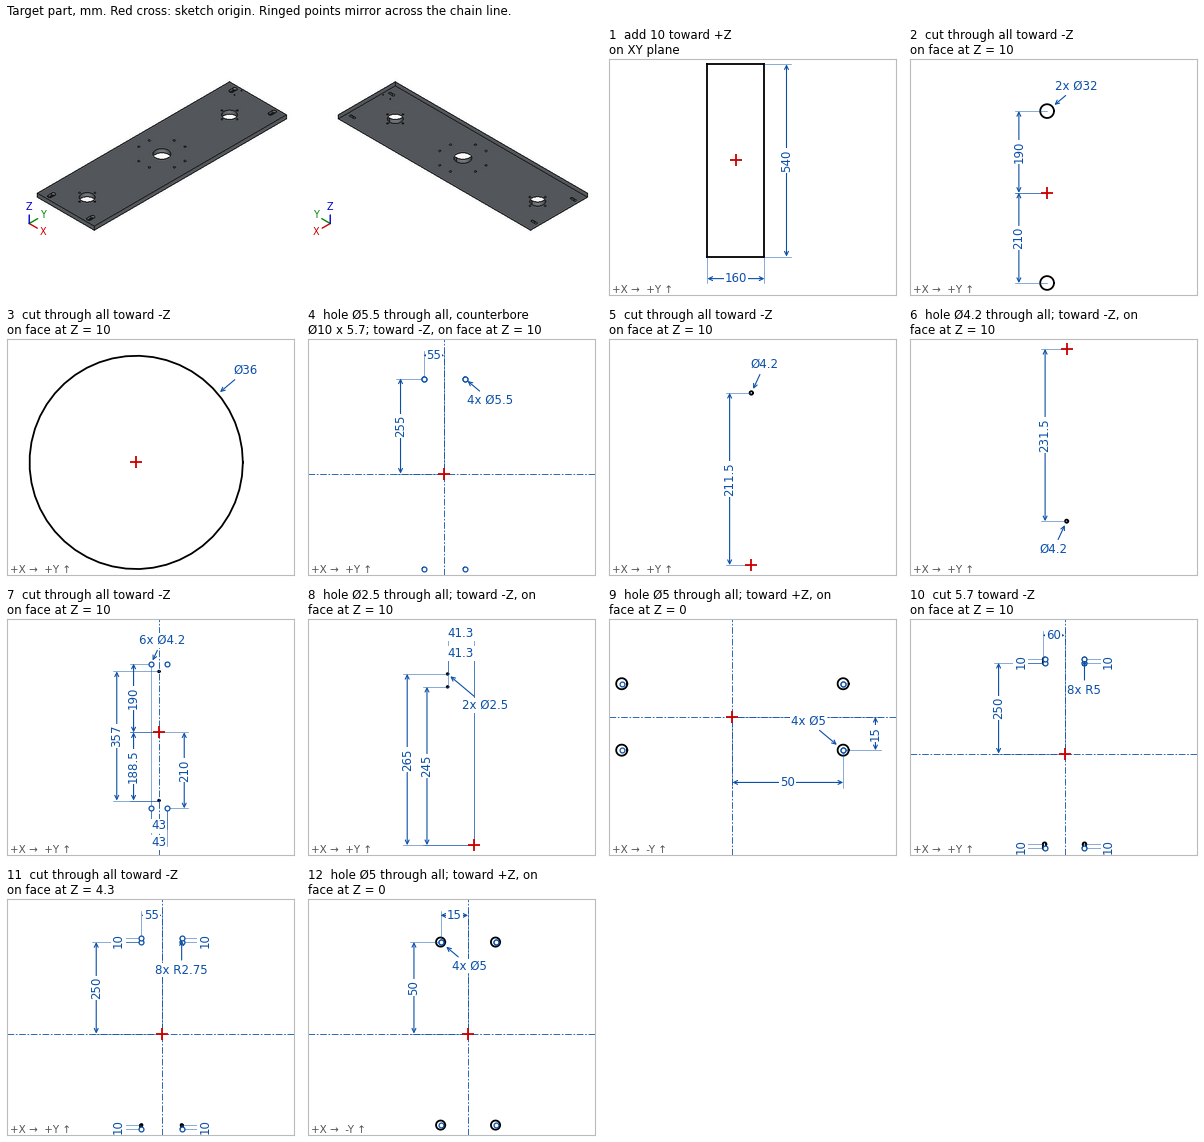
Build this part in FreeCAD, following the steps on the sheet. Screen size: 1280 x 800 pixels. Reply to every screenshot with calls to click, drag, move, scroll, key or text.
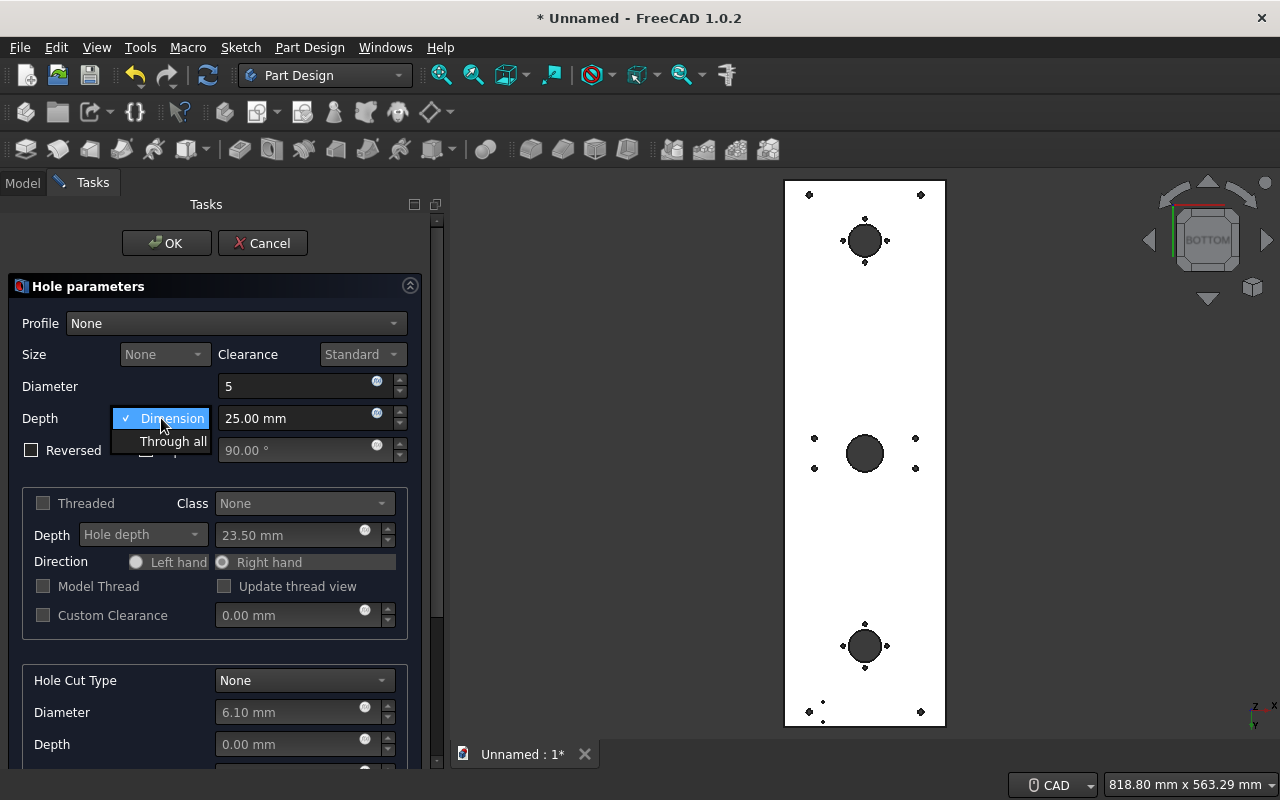
click(160, 442)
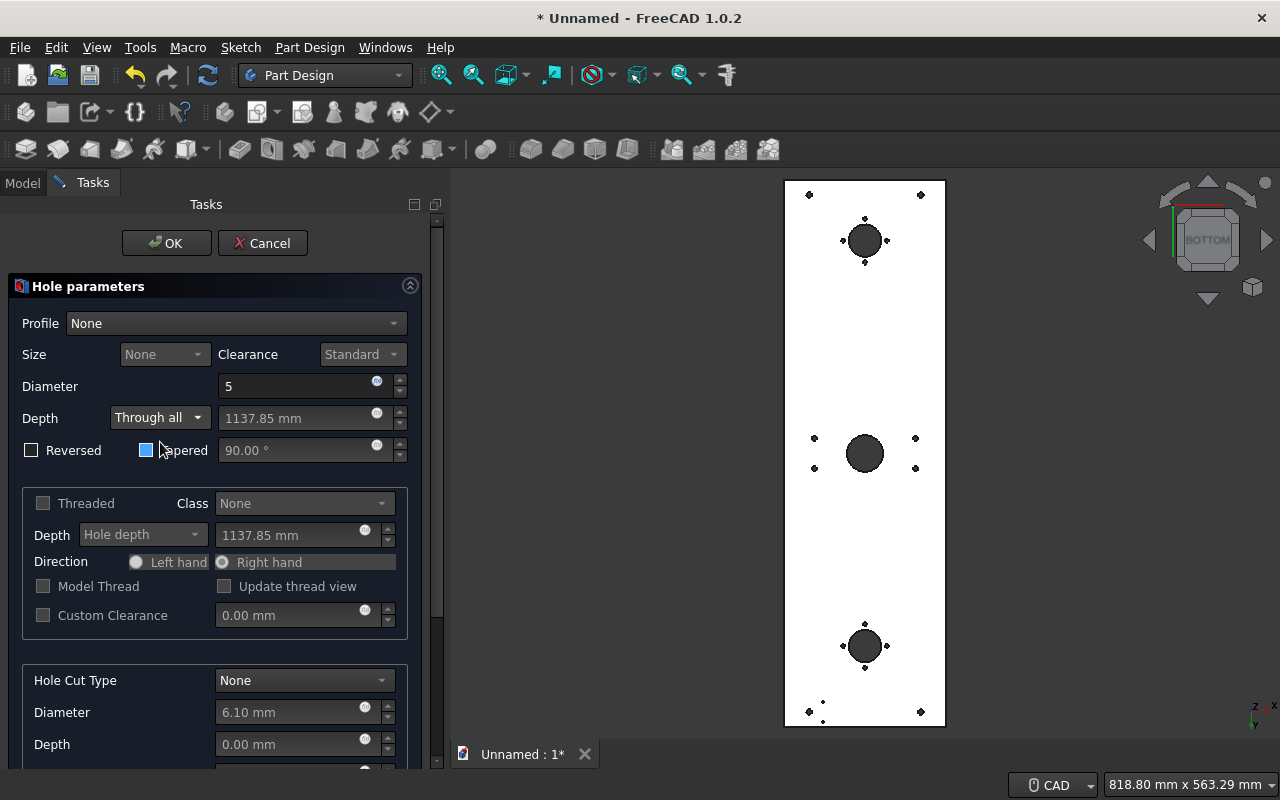
click(167, 243)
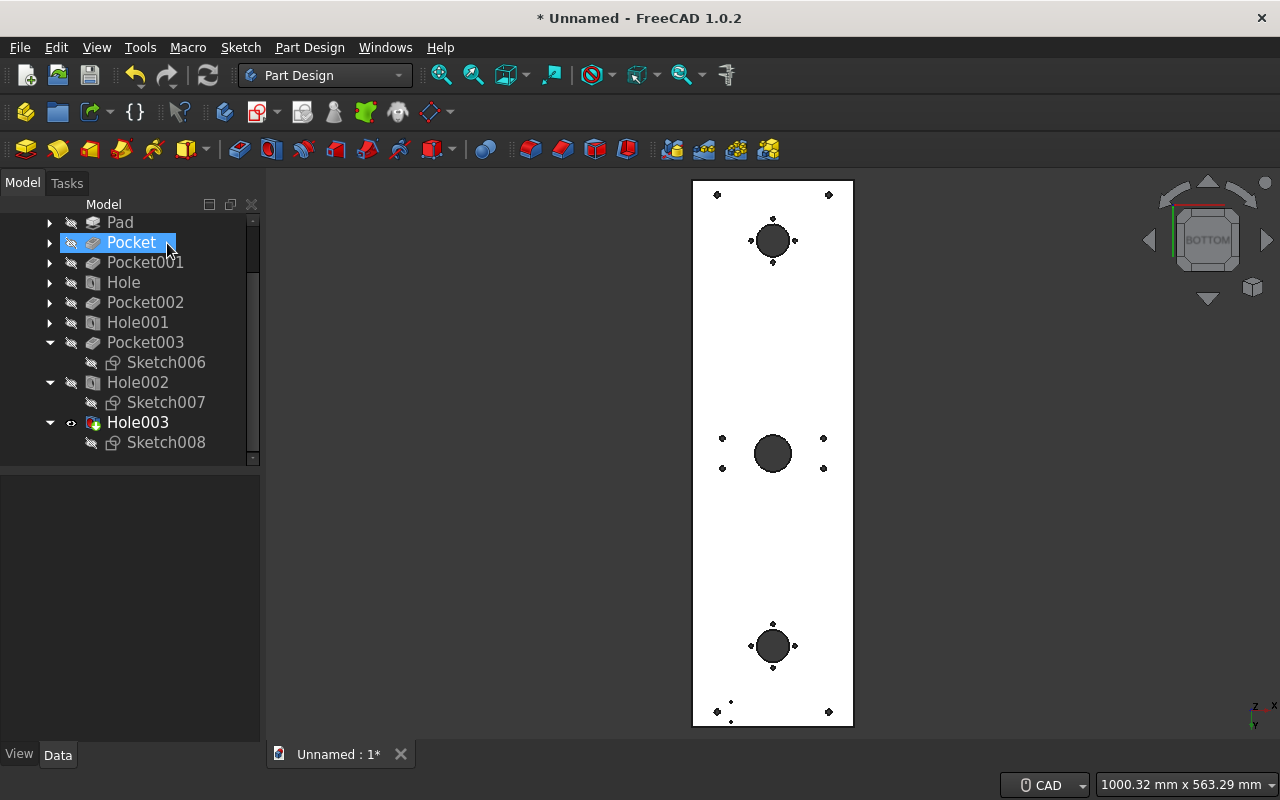
key(0)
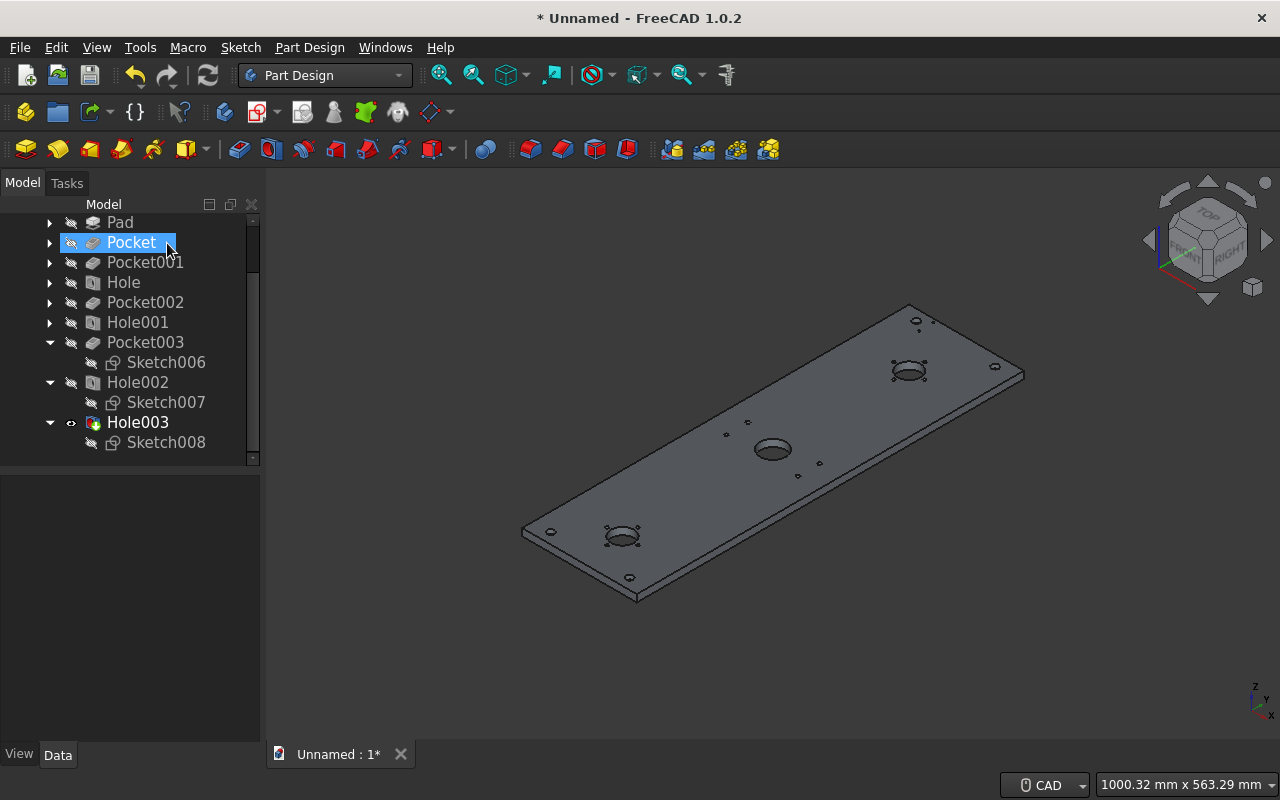
click(828, 416)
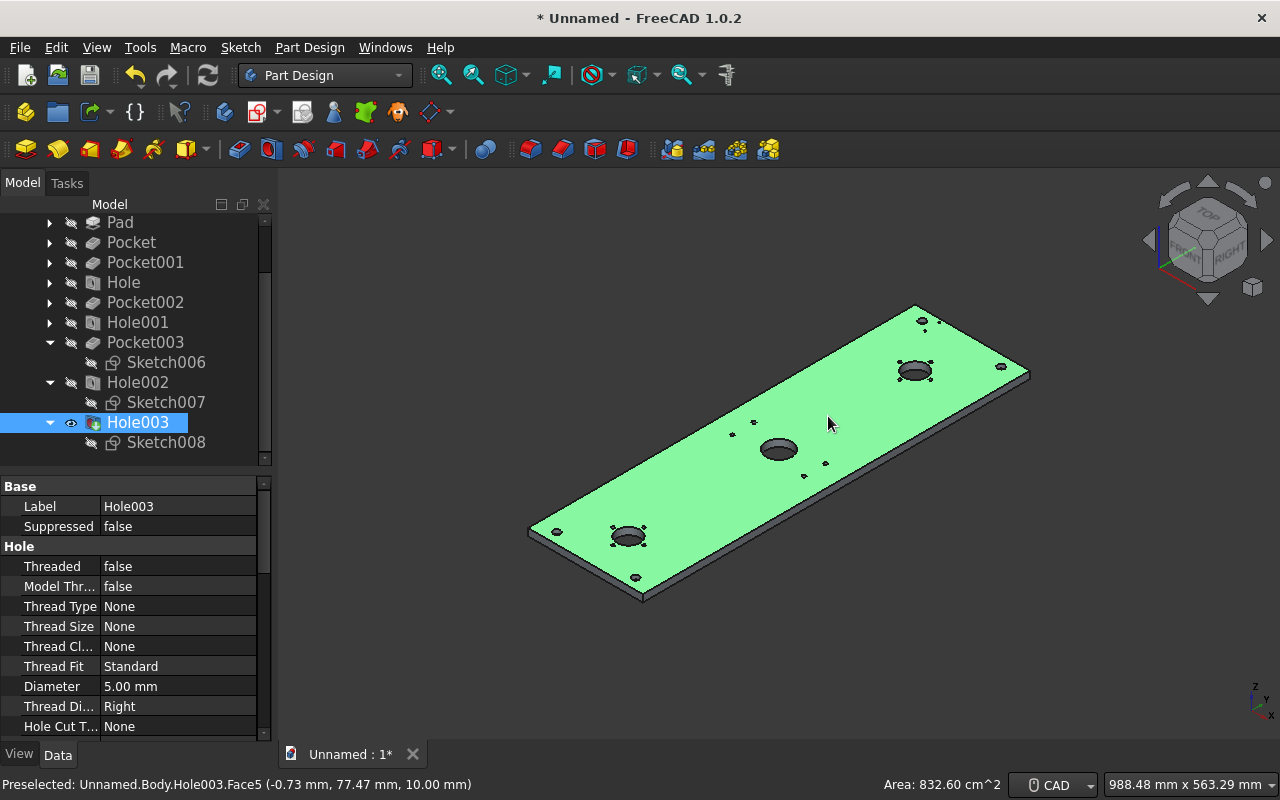
click(258, 112)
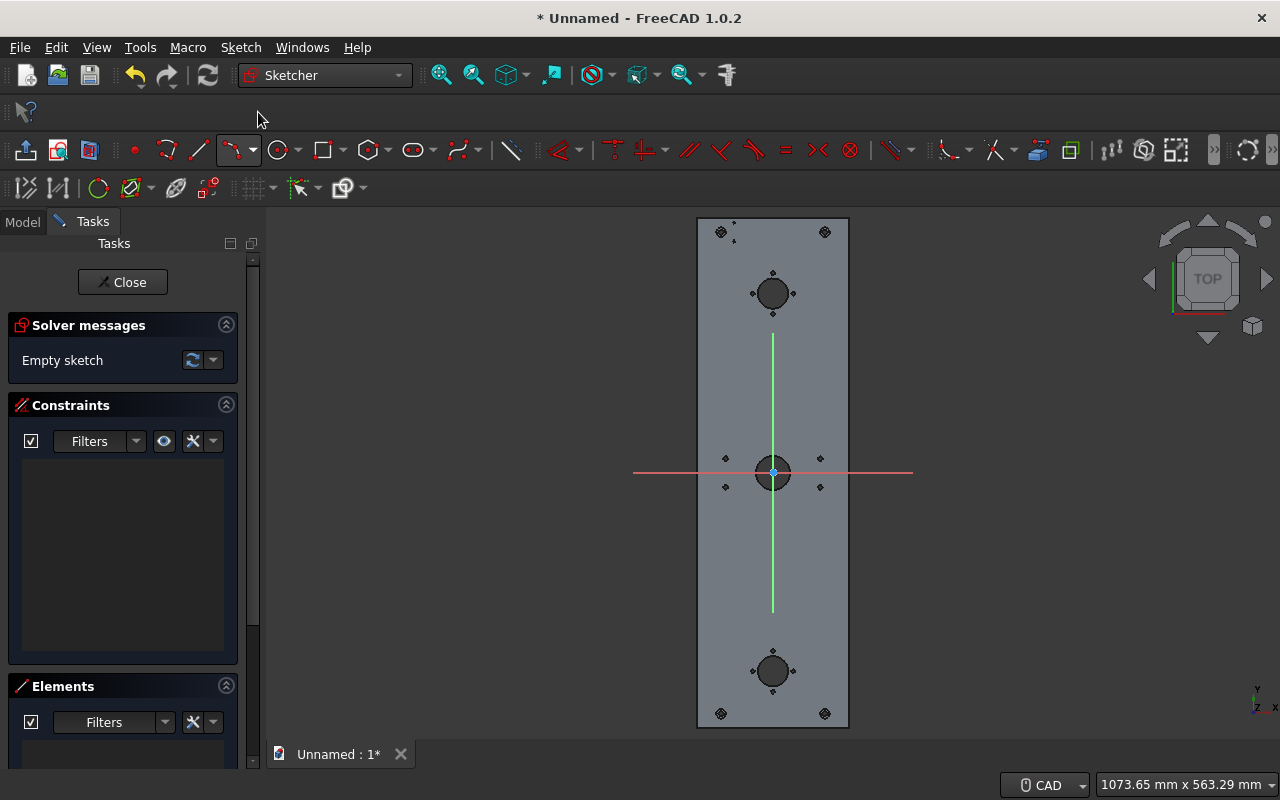
scroll(565, 473, down, 2)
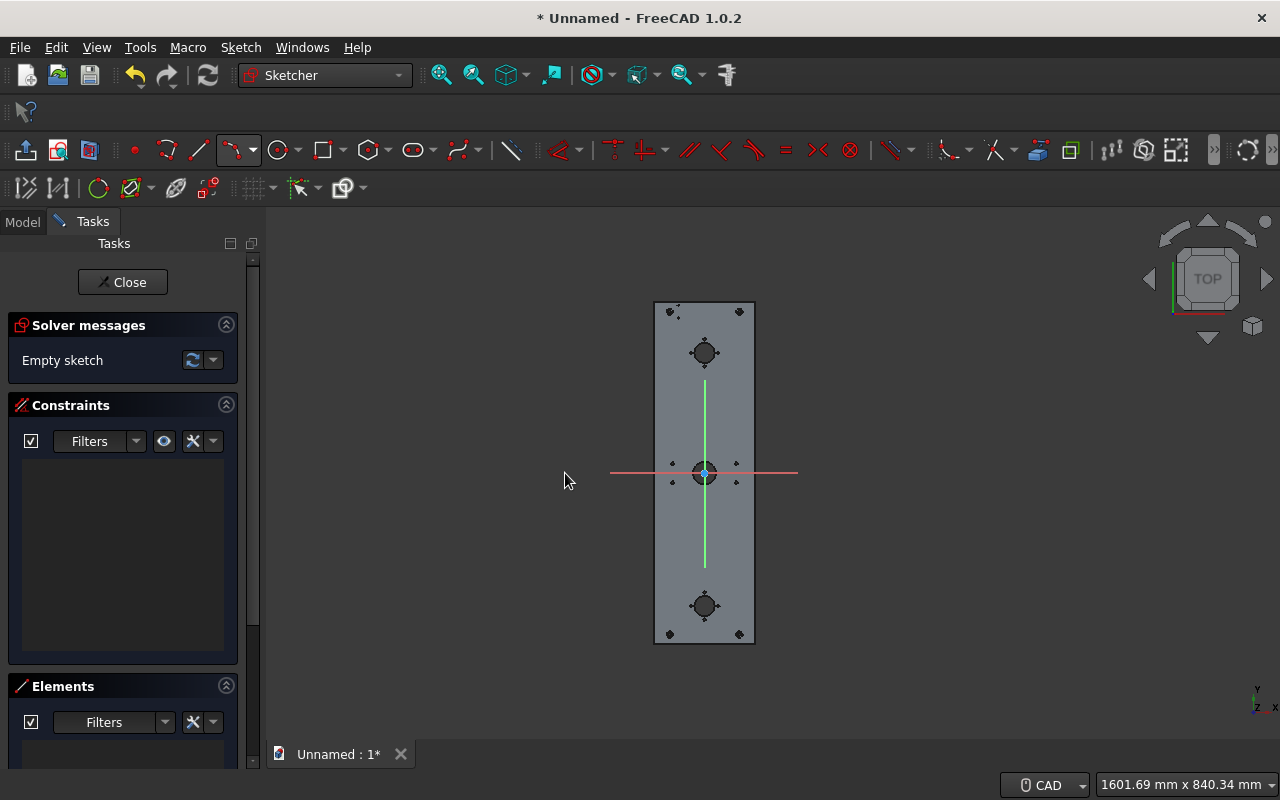
key(g)
key(s)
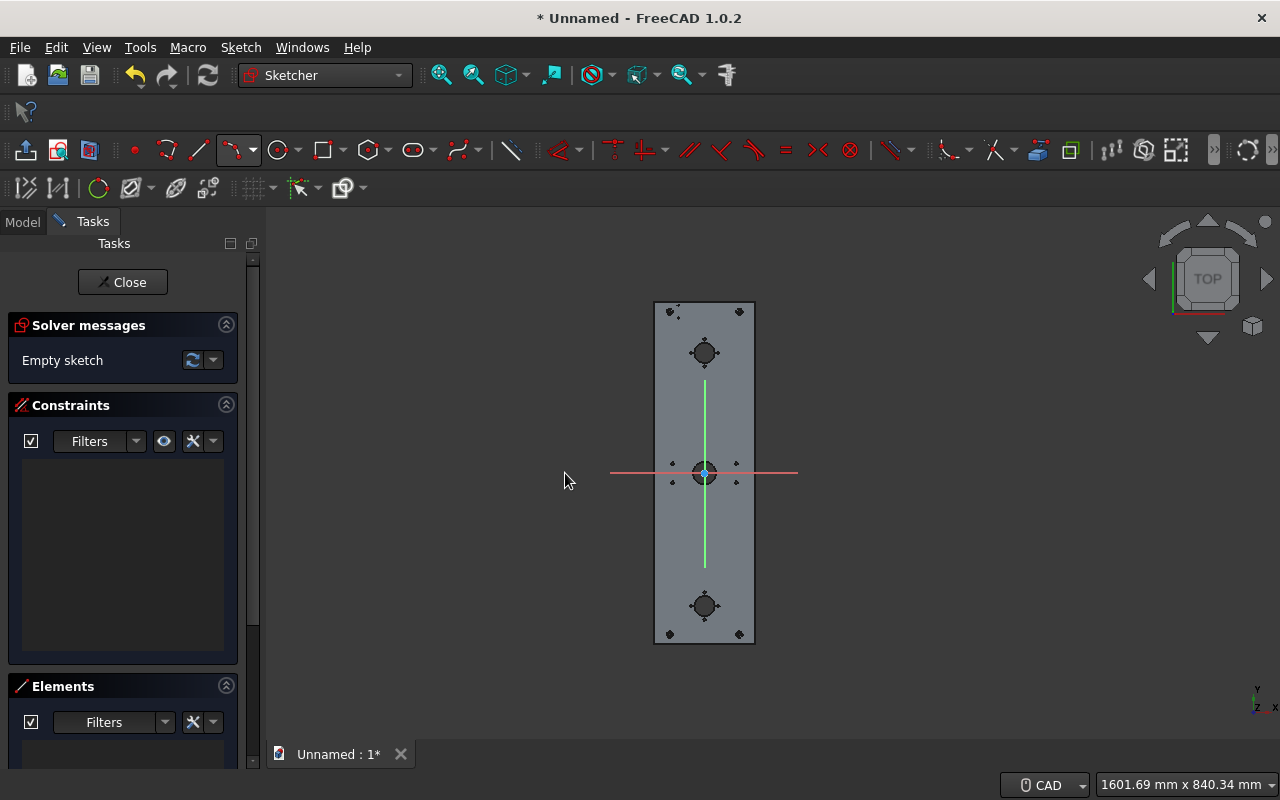
scroll(670, 315, up, 10)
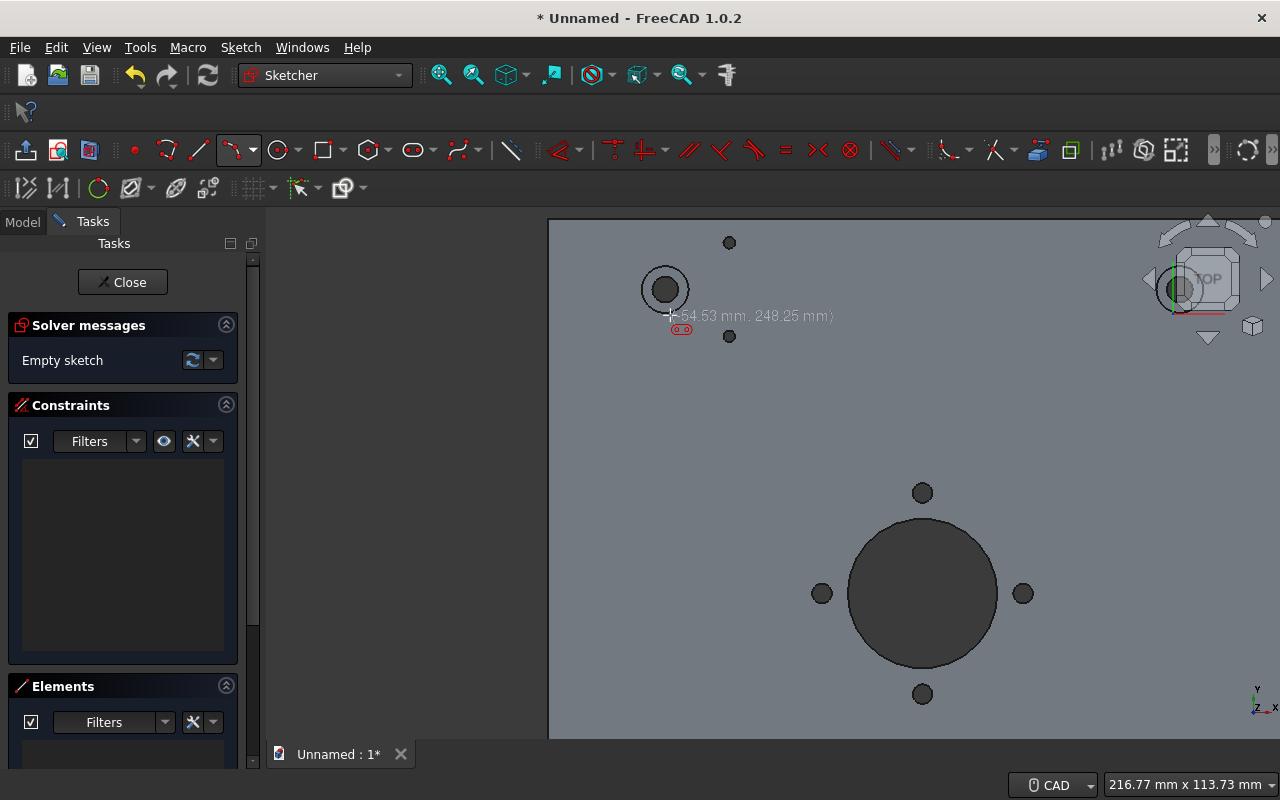
scroll(670, 315, down, 10)